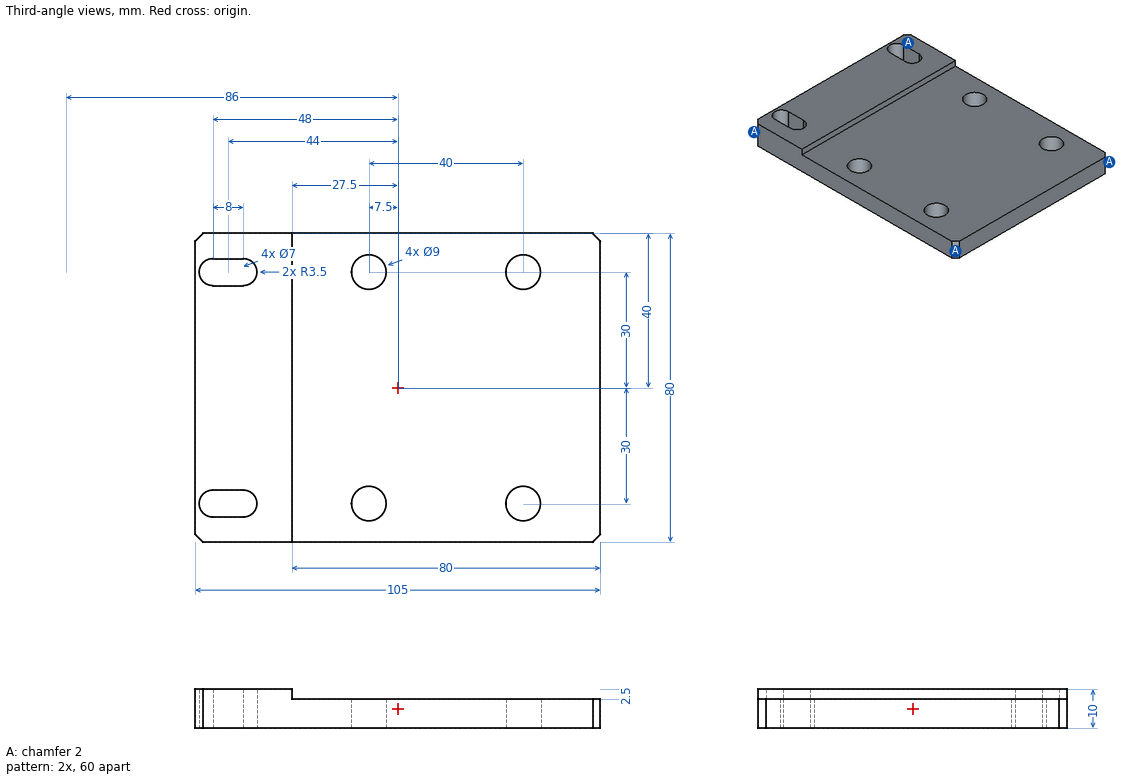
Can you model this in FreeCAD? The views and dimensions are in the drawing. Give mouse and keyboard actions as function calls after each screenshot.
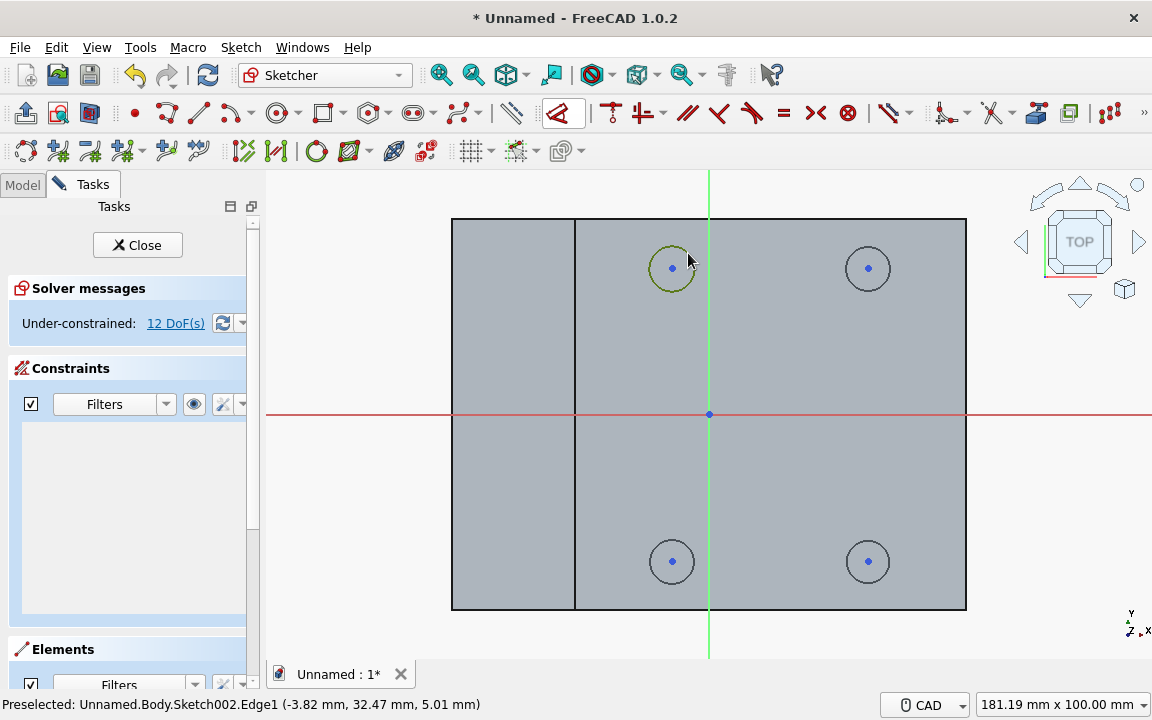
click(883, 253)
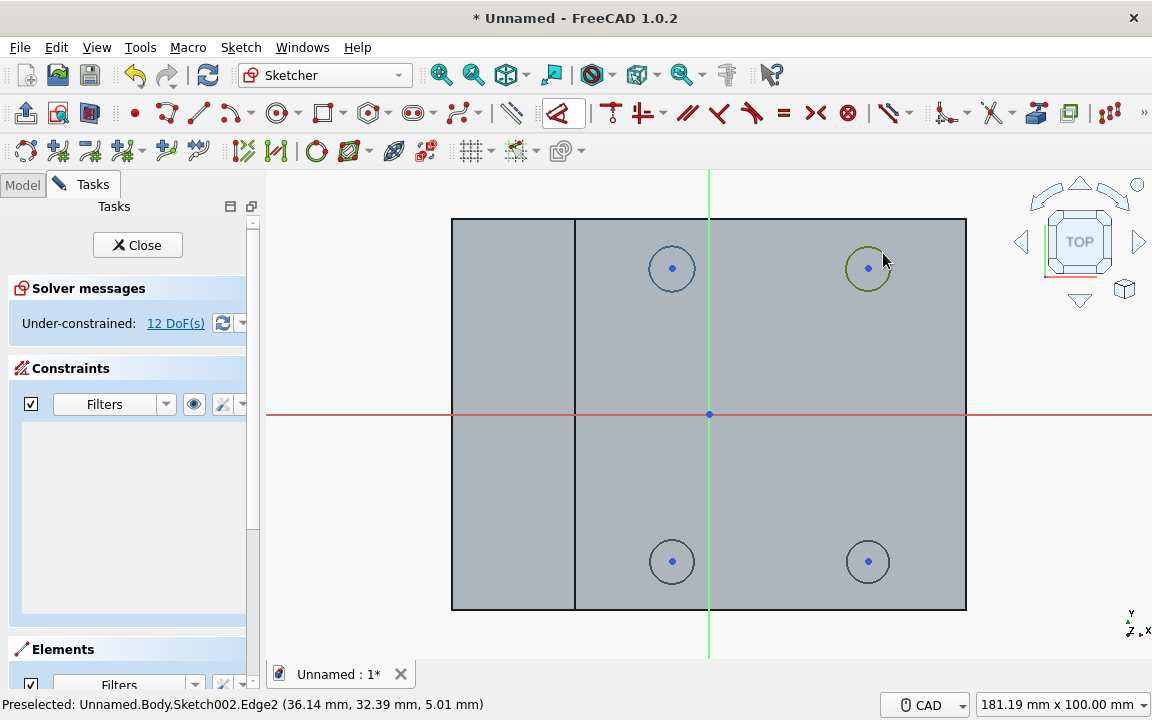
click(883, 547)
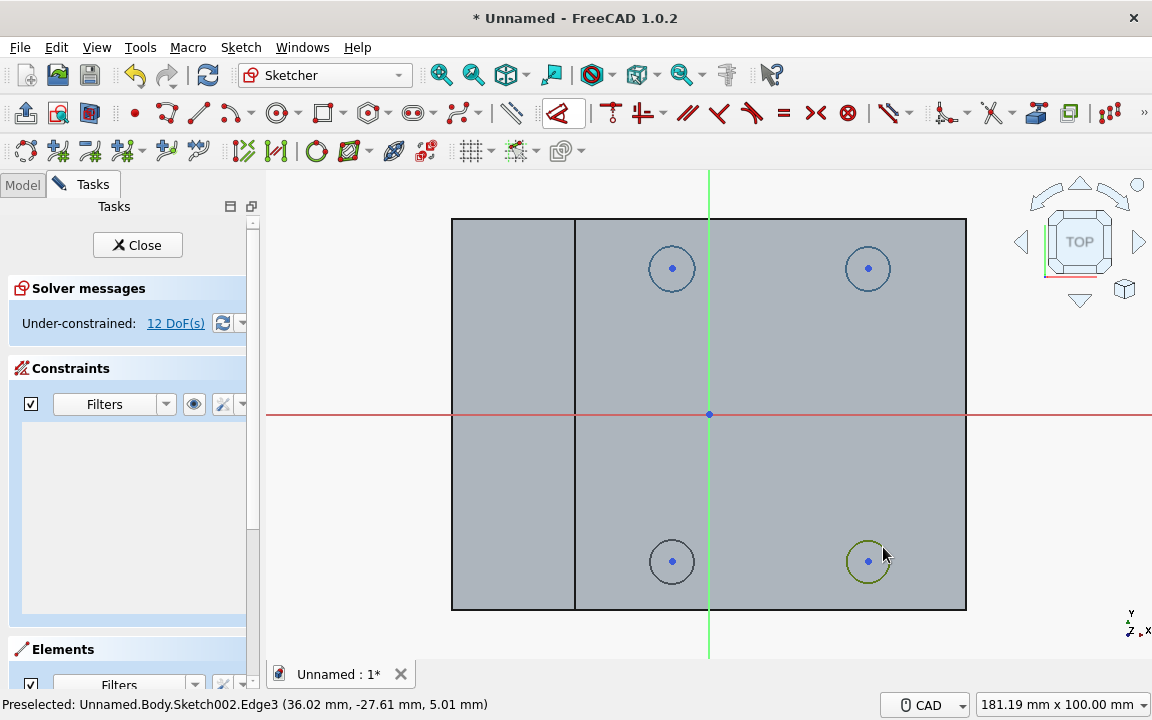
click(687, 546)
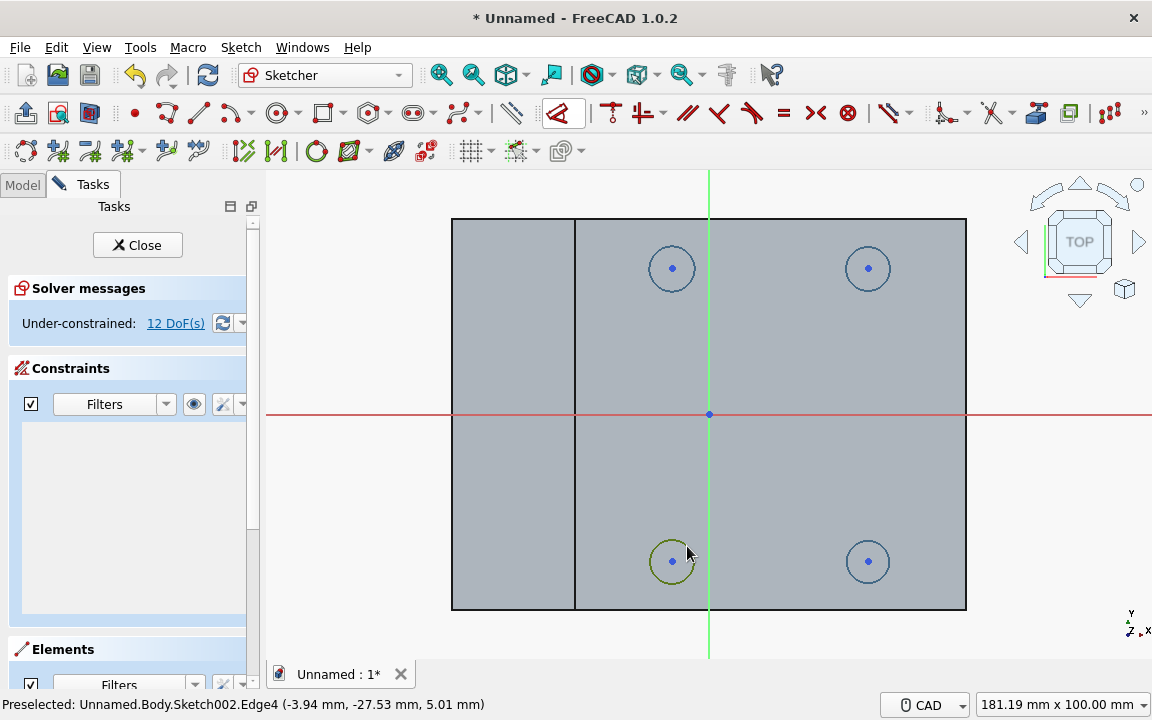
click(784, 114)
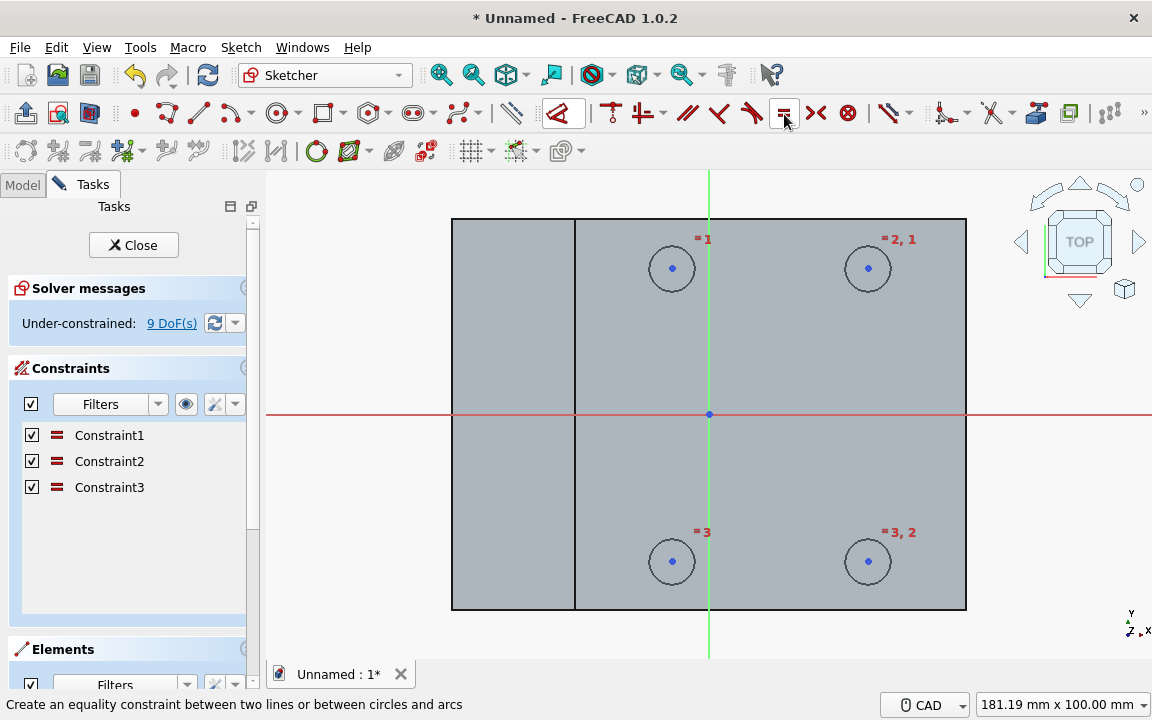
click(672, 269)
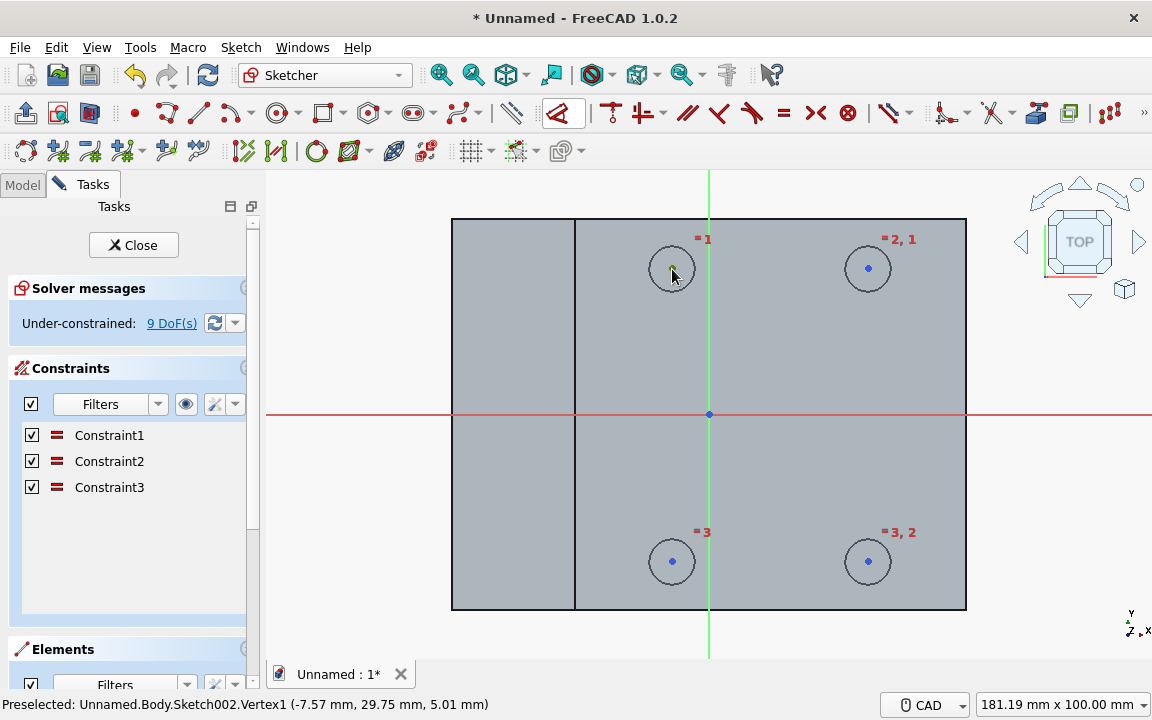
click(868, 269)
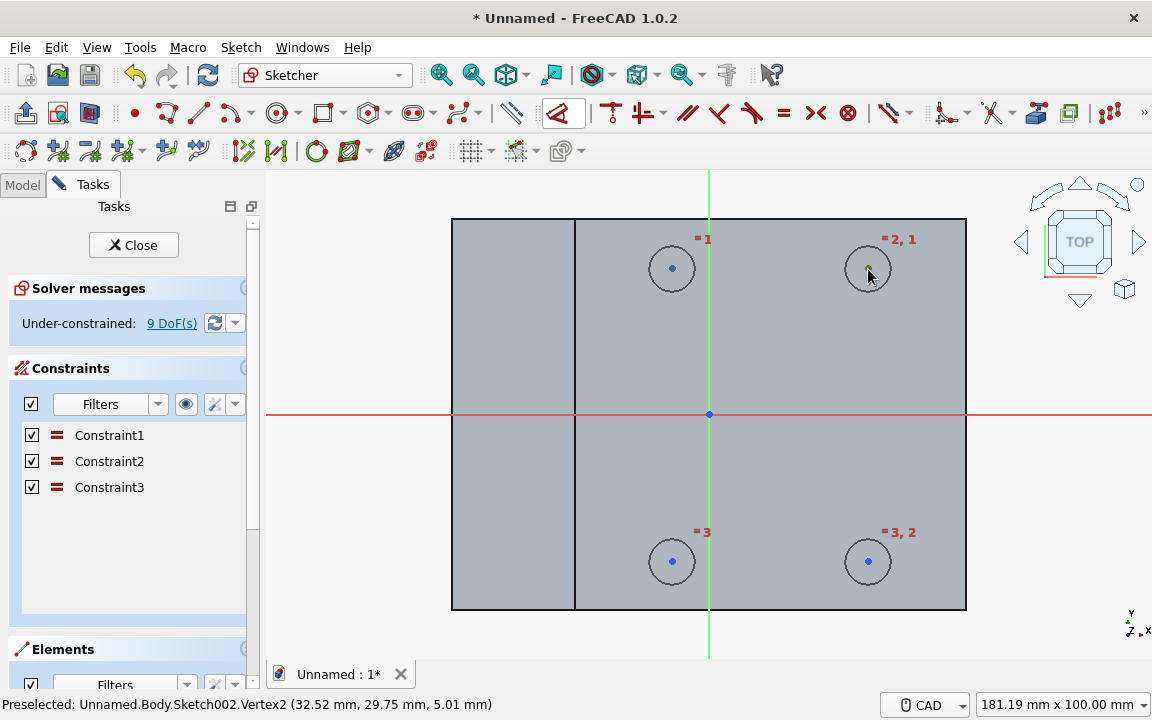
key(h)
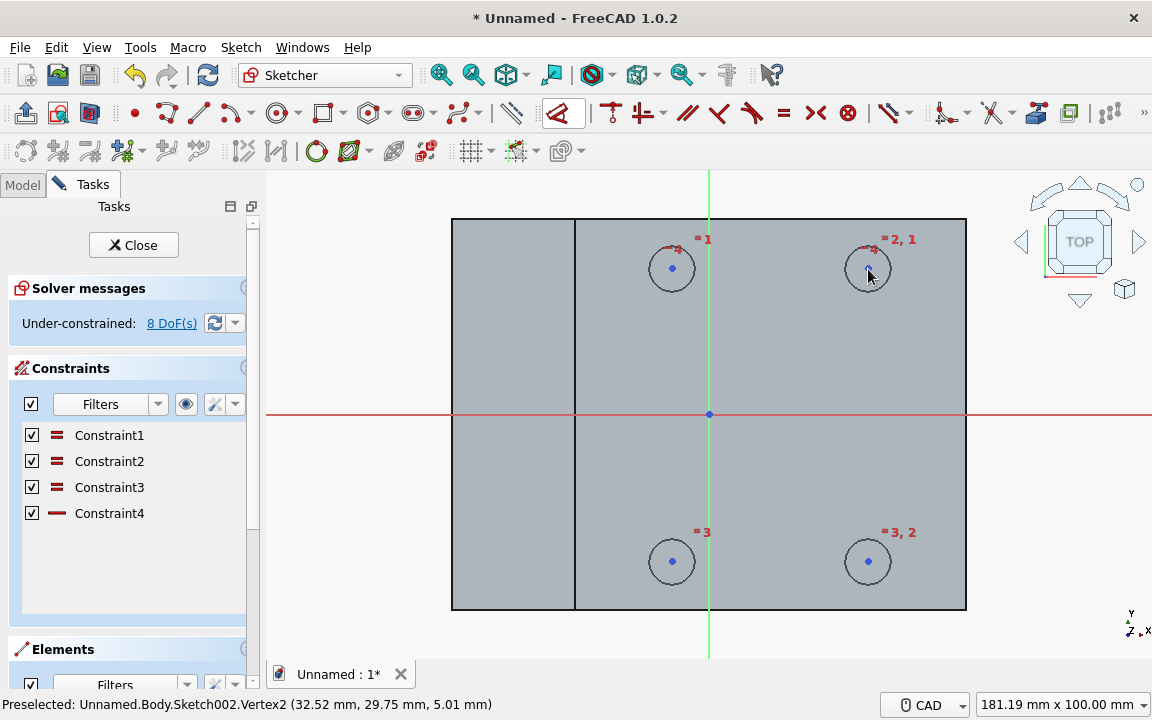
click(868, 269)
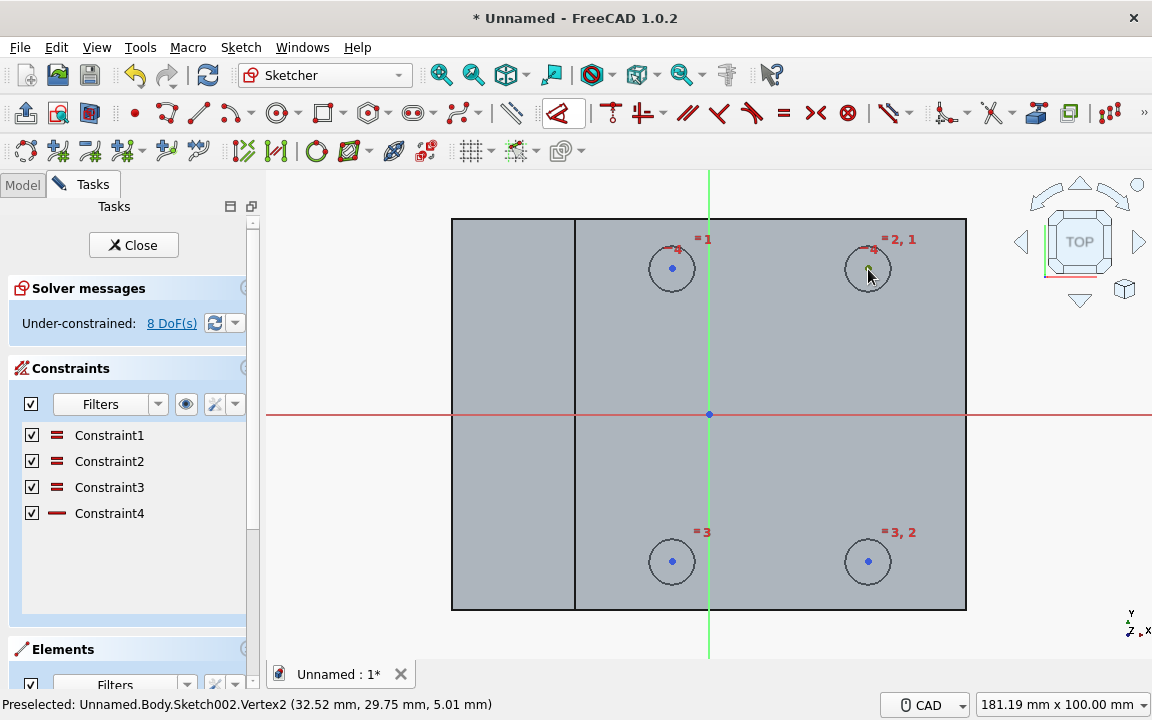
click(868, 562)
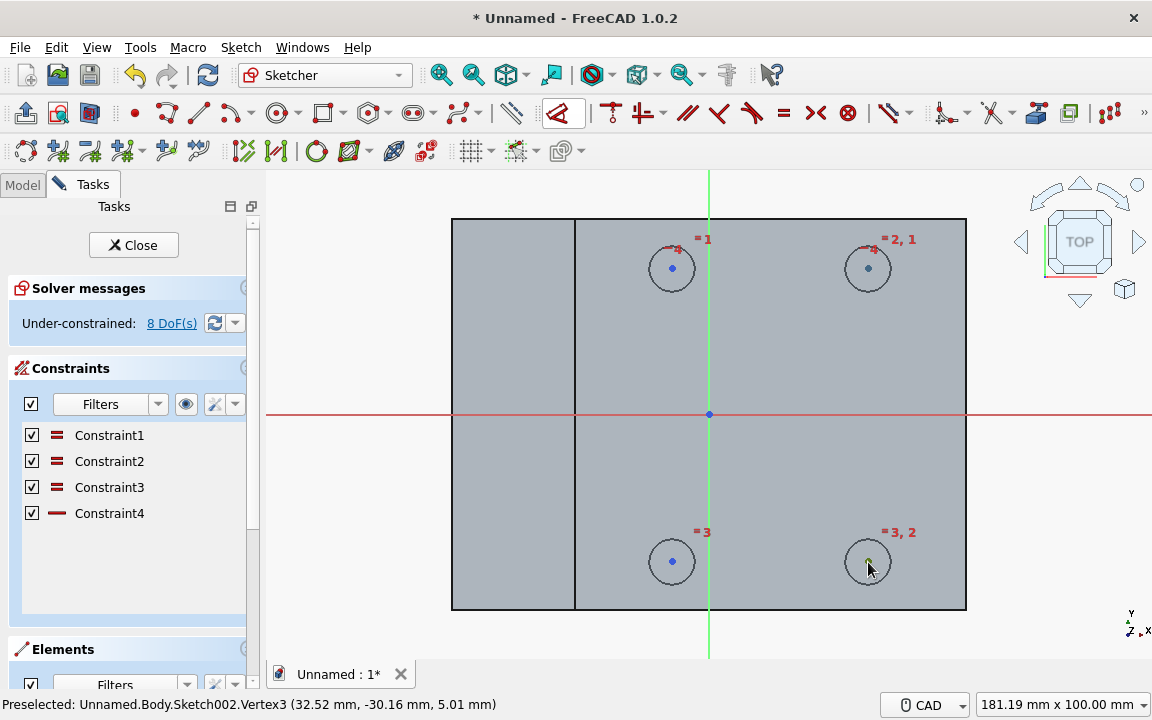
click(666, 114)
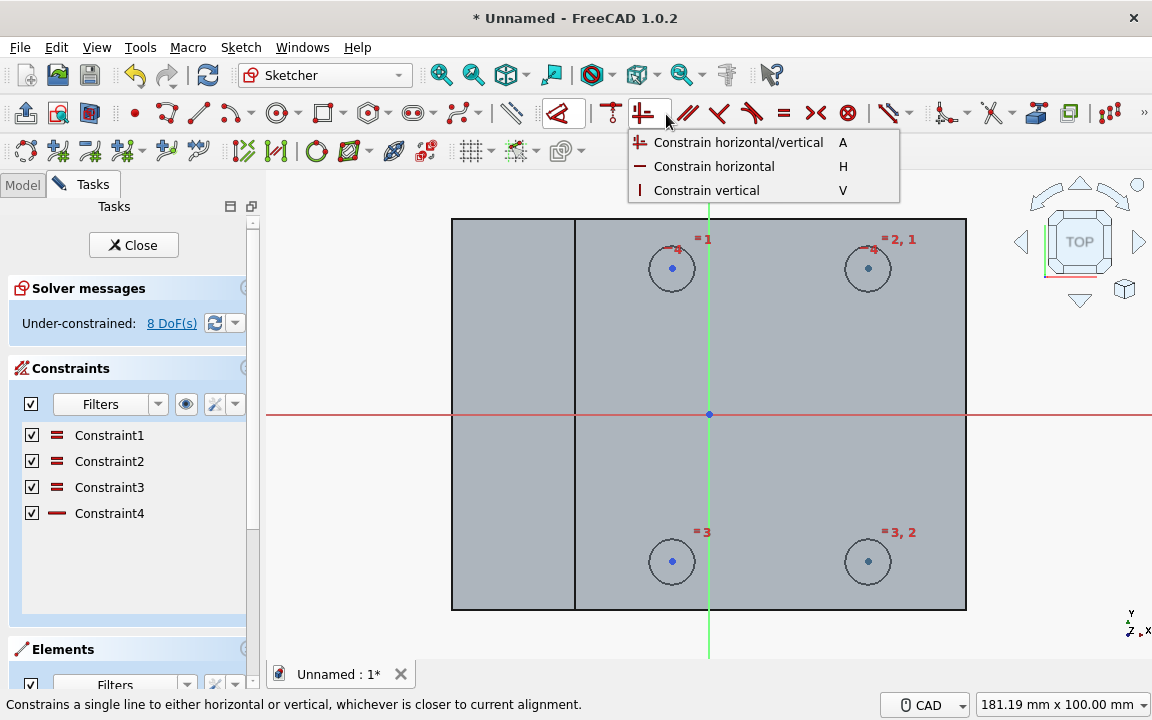
click(764, 190)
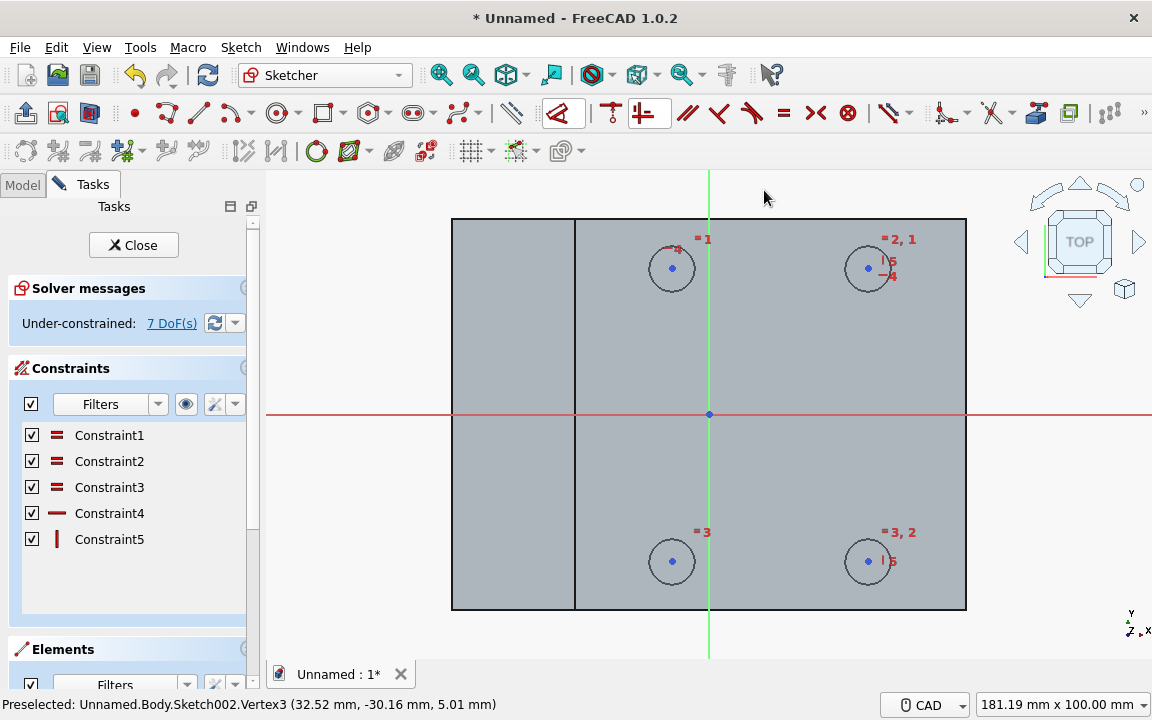
click(672, 269)